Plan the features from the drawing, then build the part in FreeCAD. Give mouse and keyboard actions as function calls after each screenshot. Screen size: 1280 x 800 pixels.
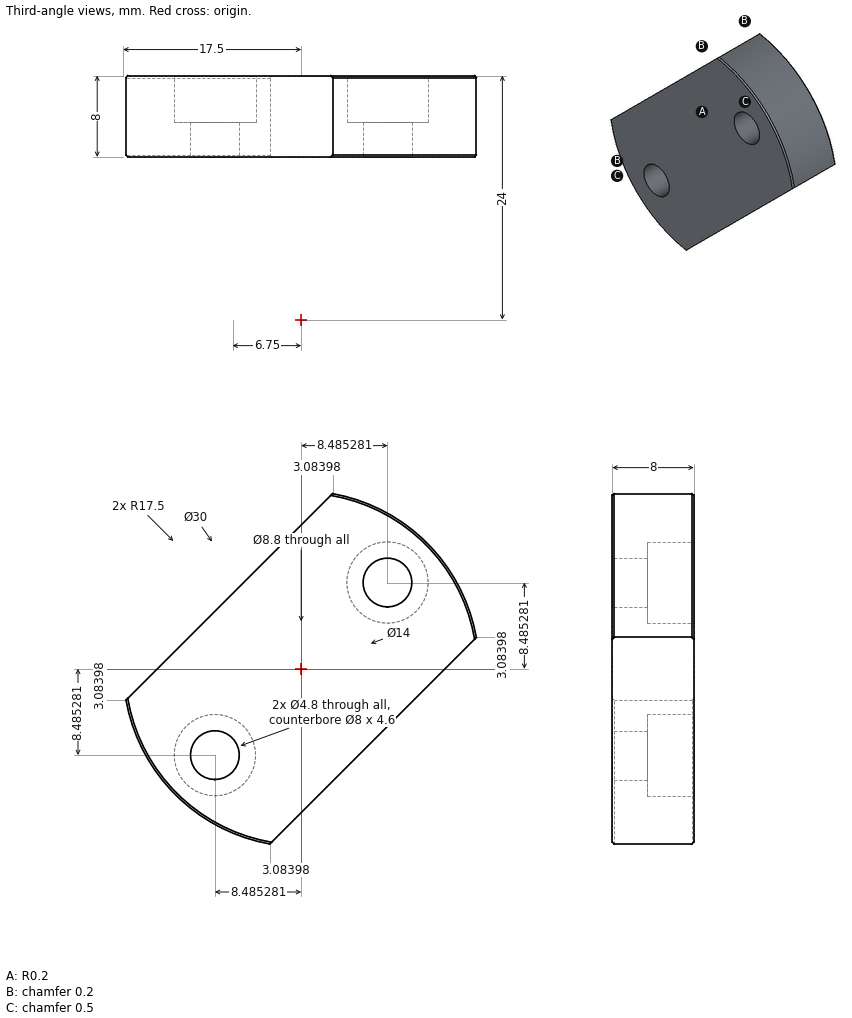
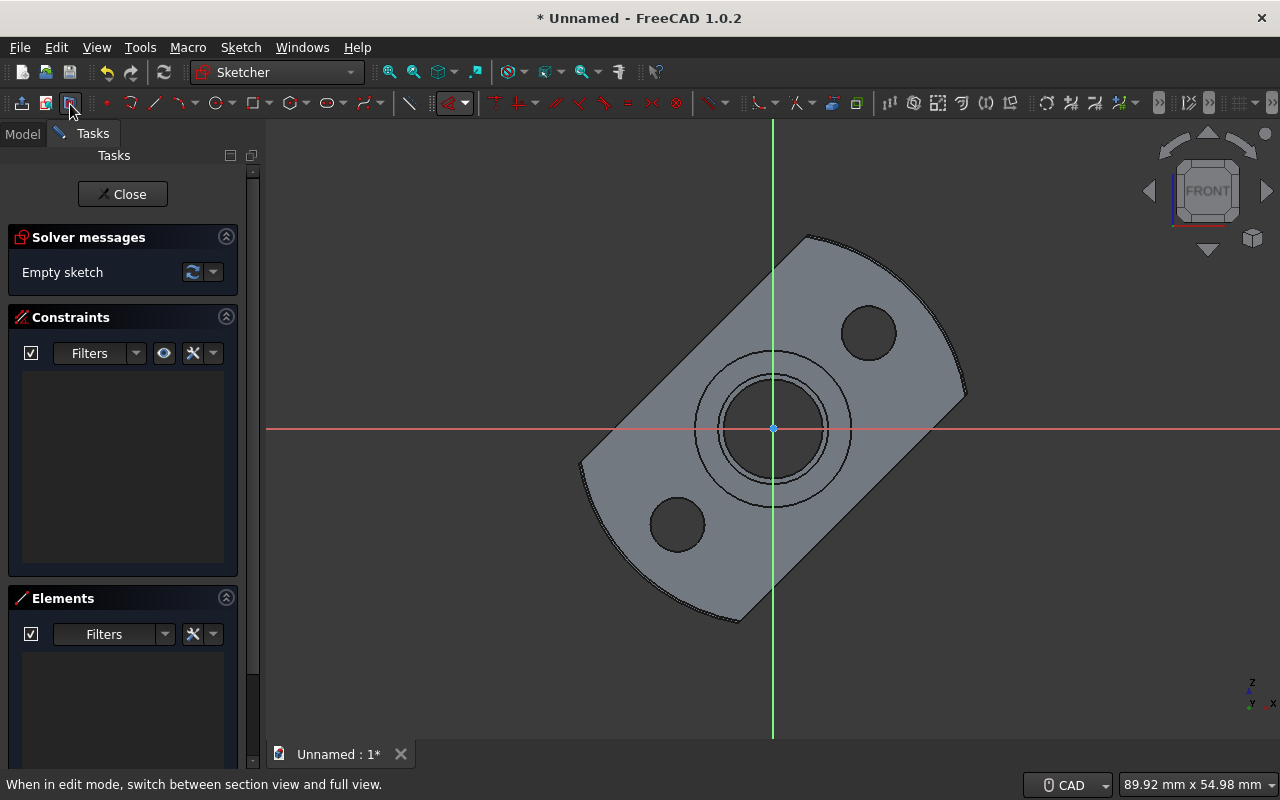
click(216, 104)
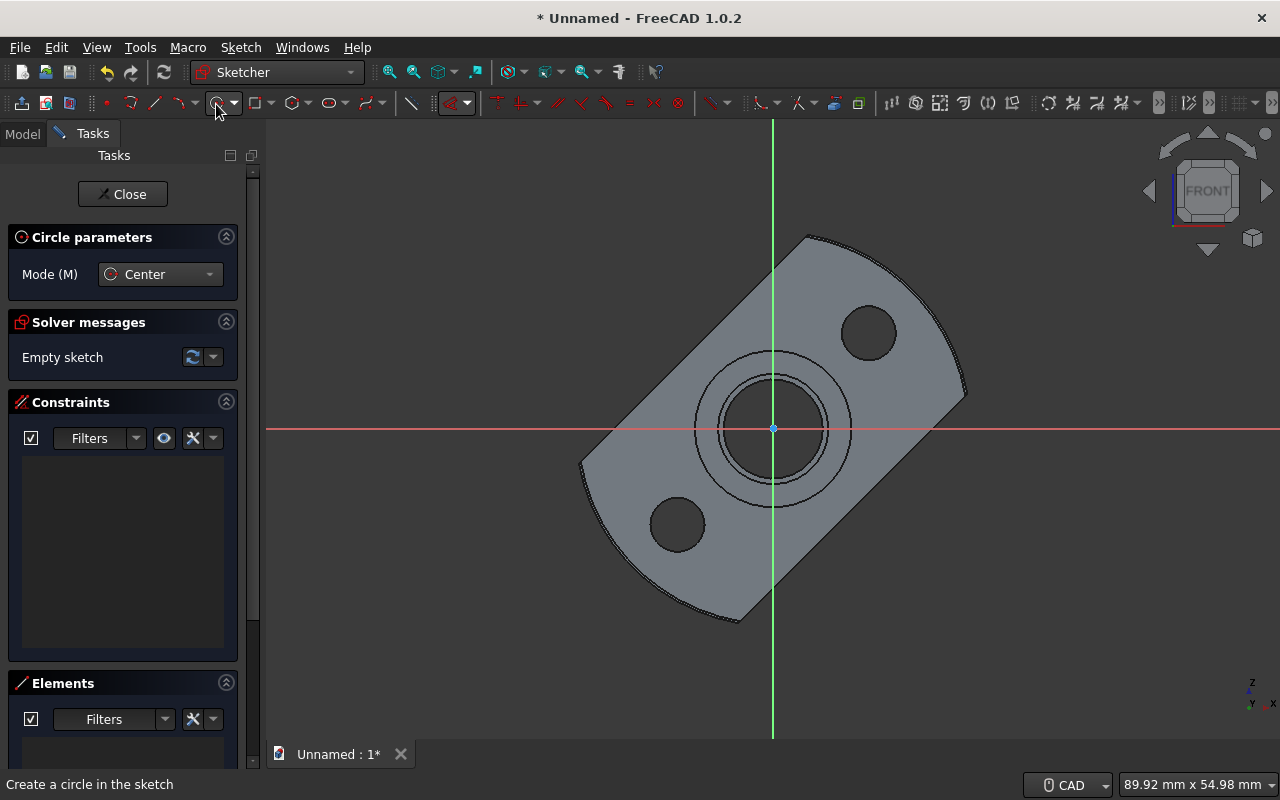
click(773, 429)
move(893, 309)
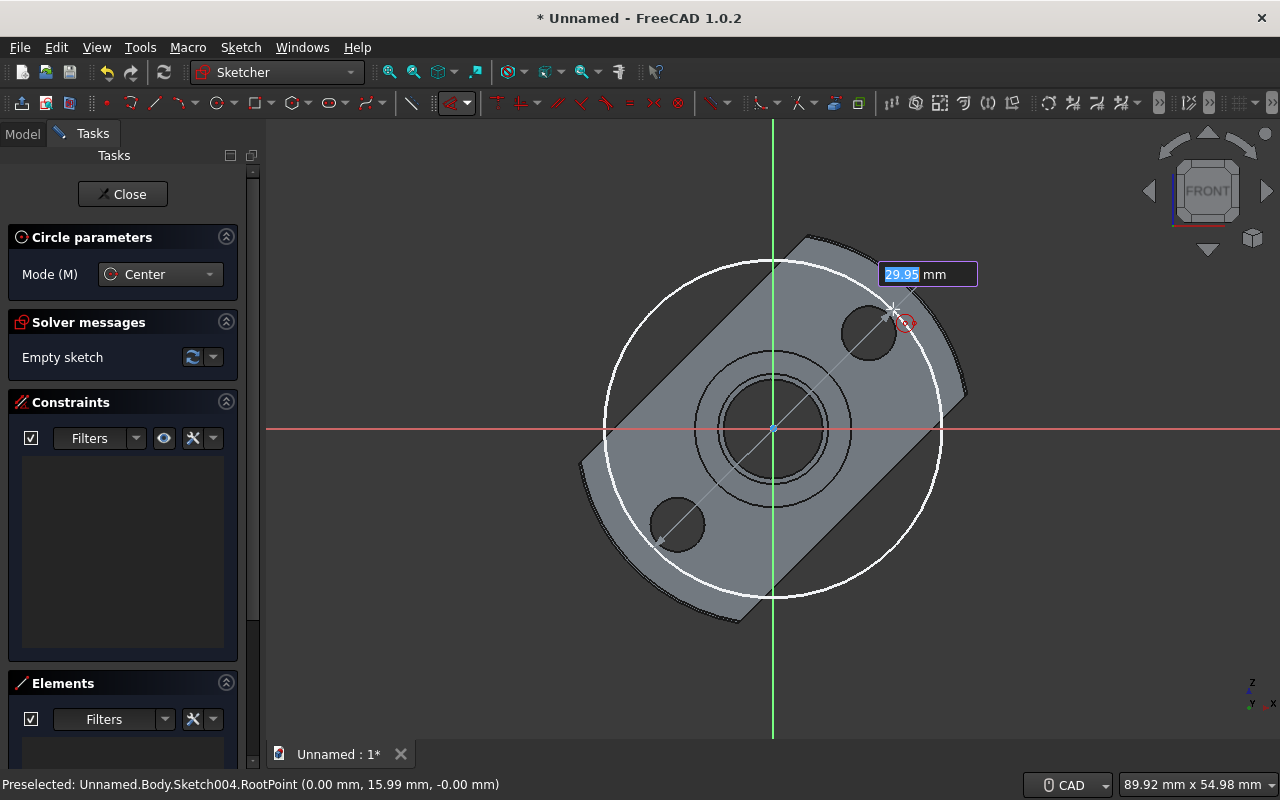
text(30)
key(Return)
key(Escape)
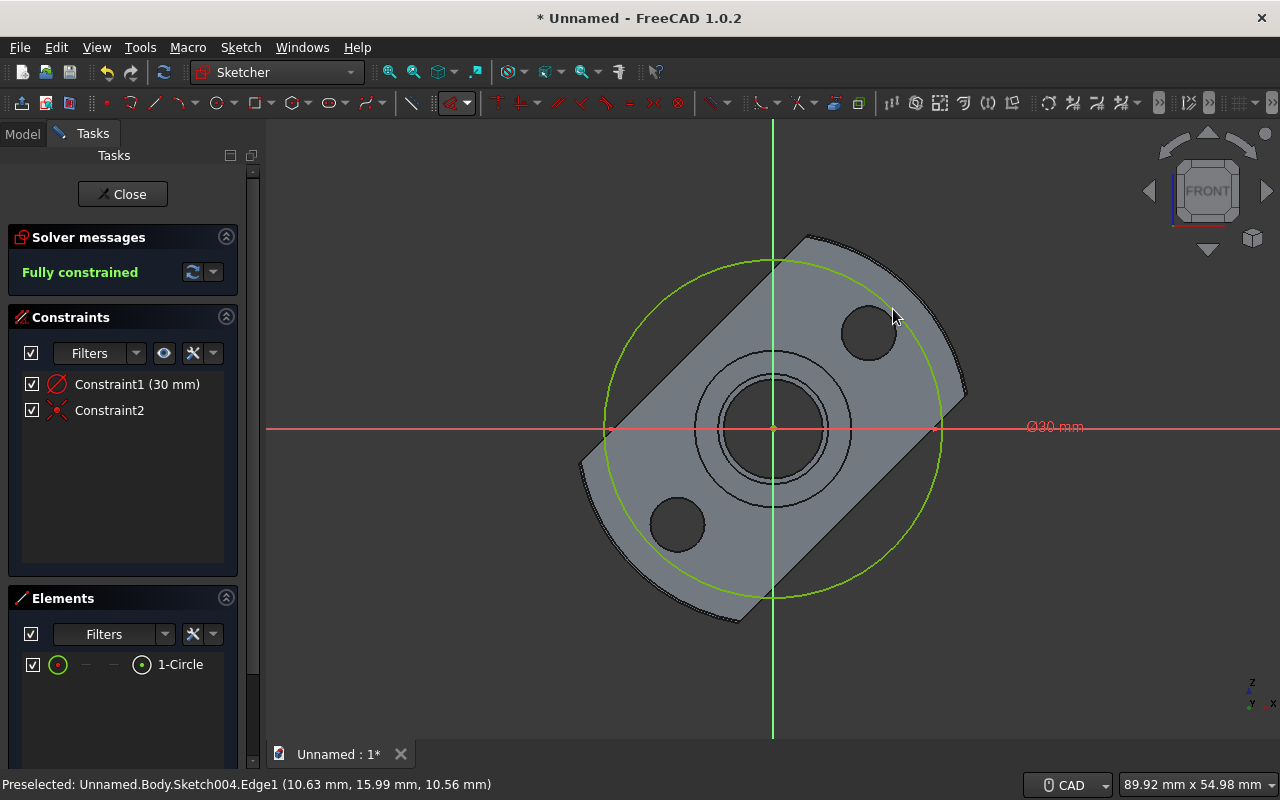
click(123, 194)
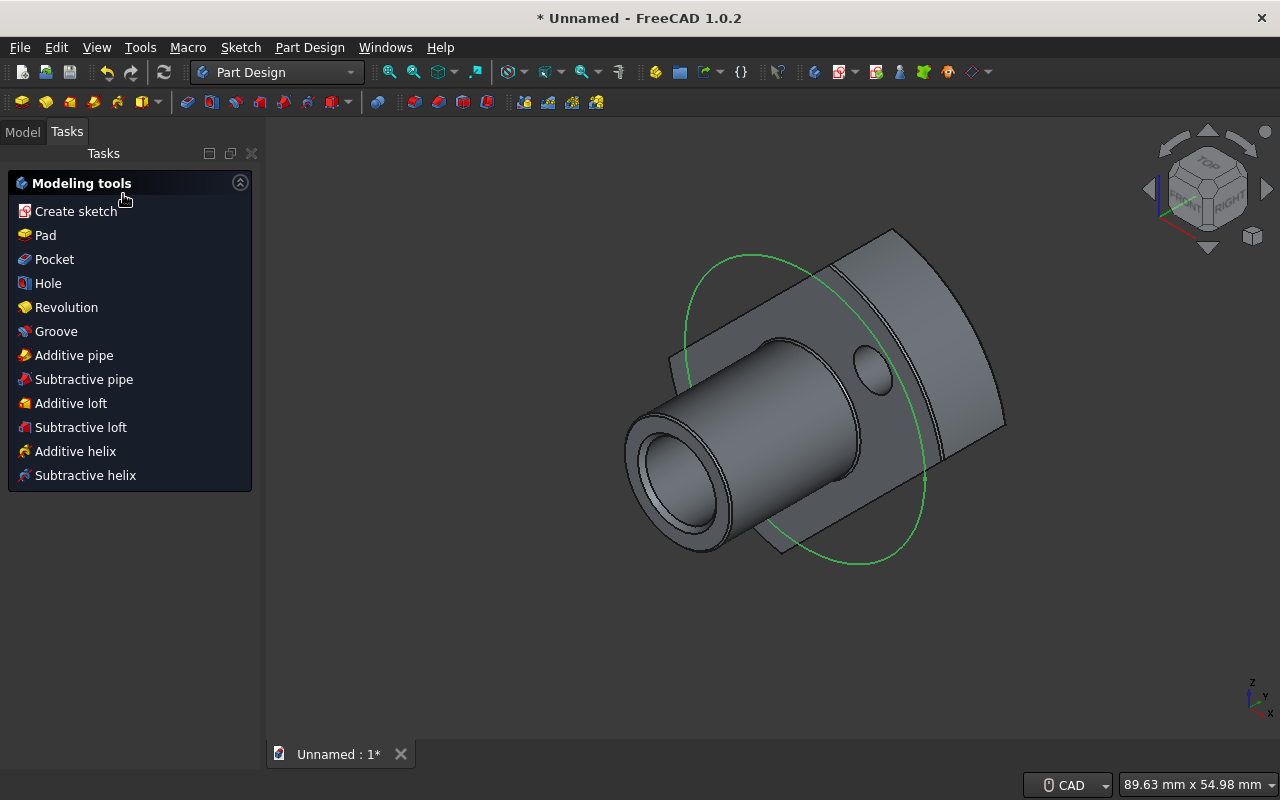
click(188, 102)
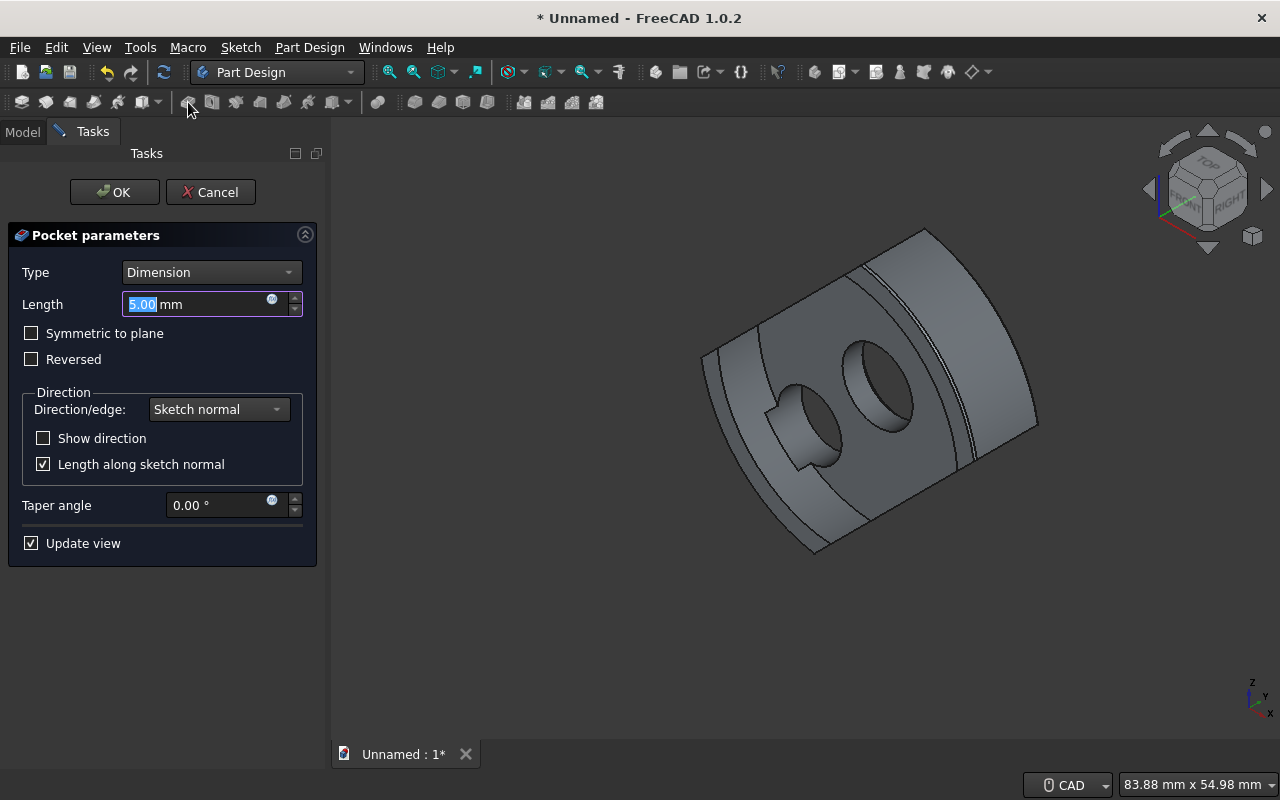
click(212, 272)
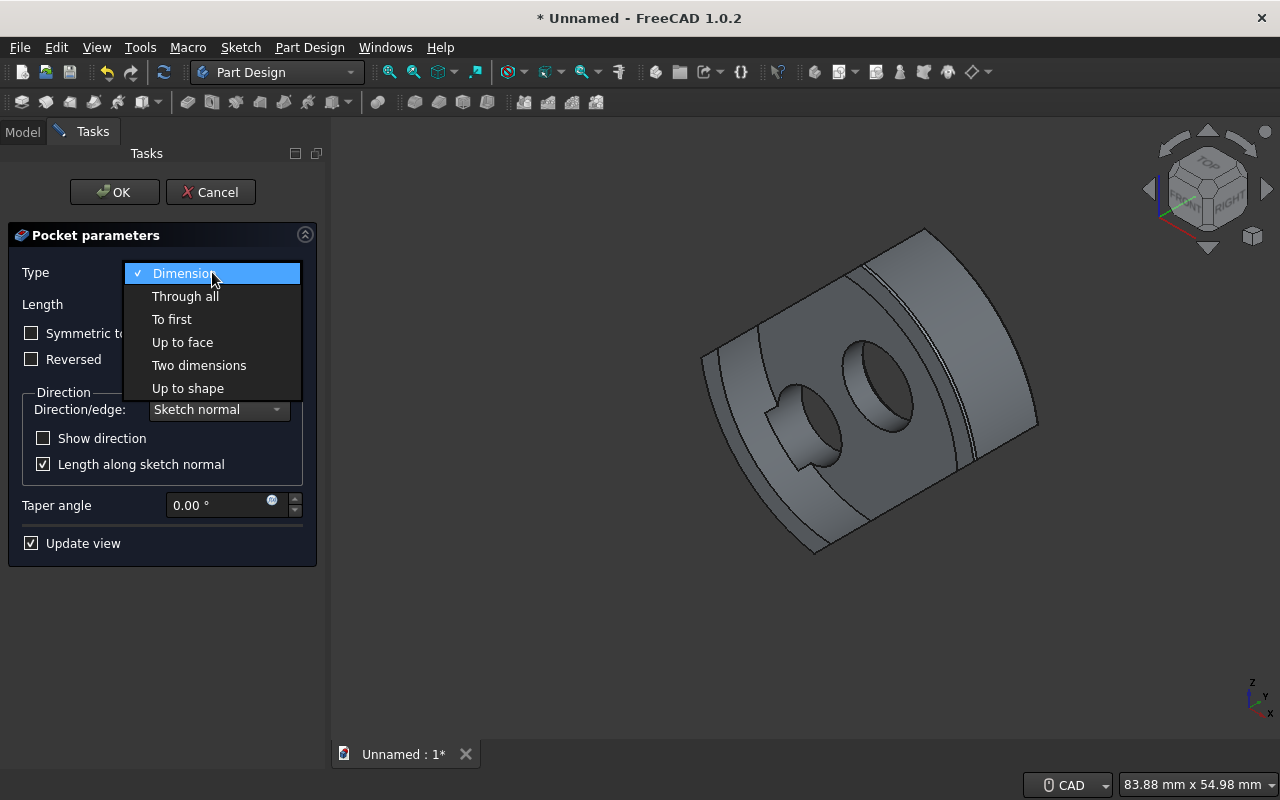
click(212, 296)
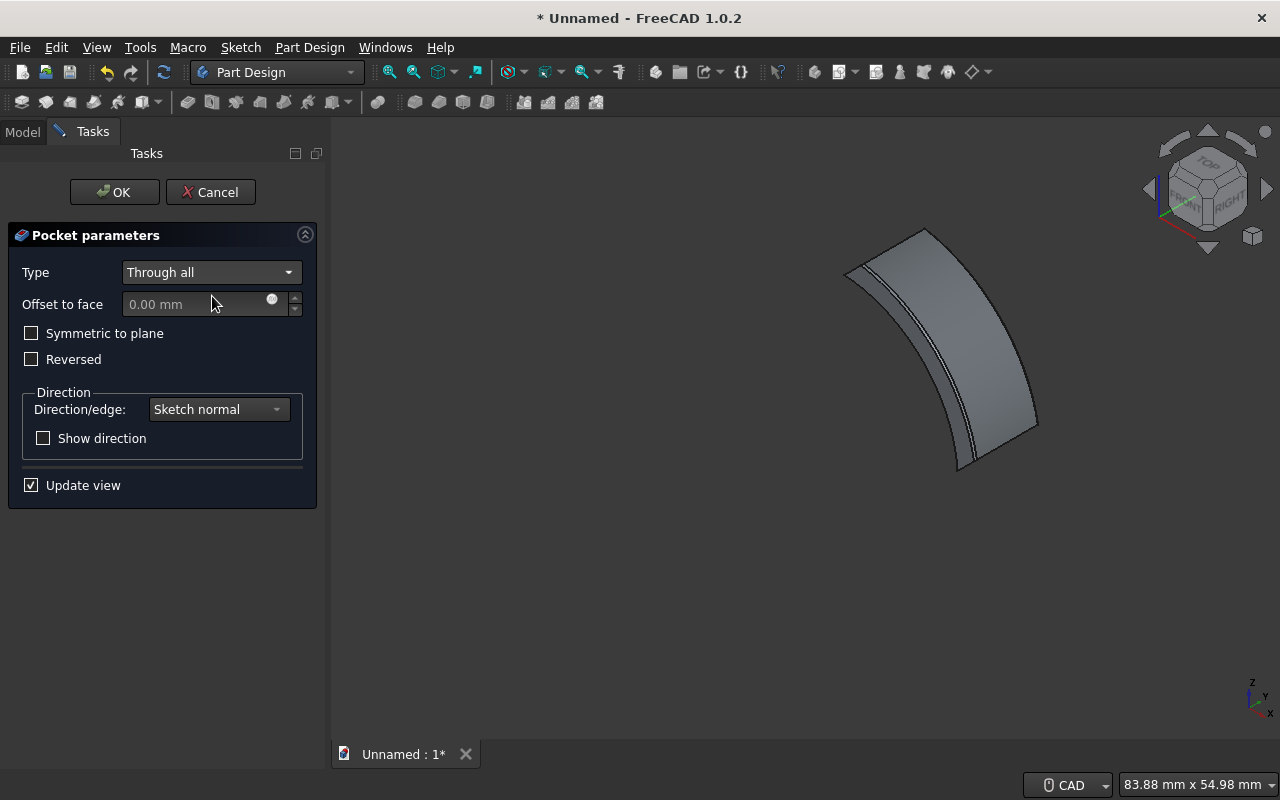
click(30, 359)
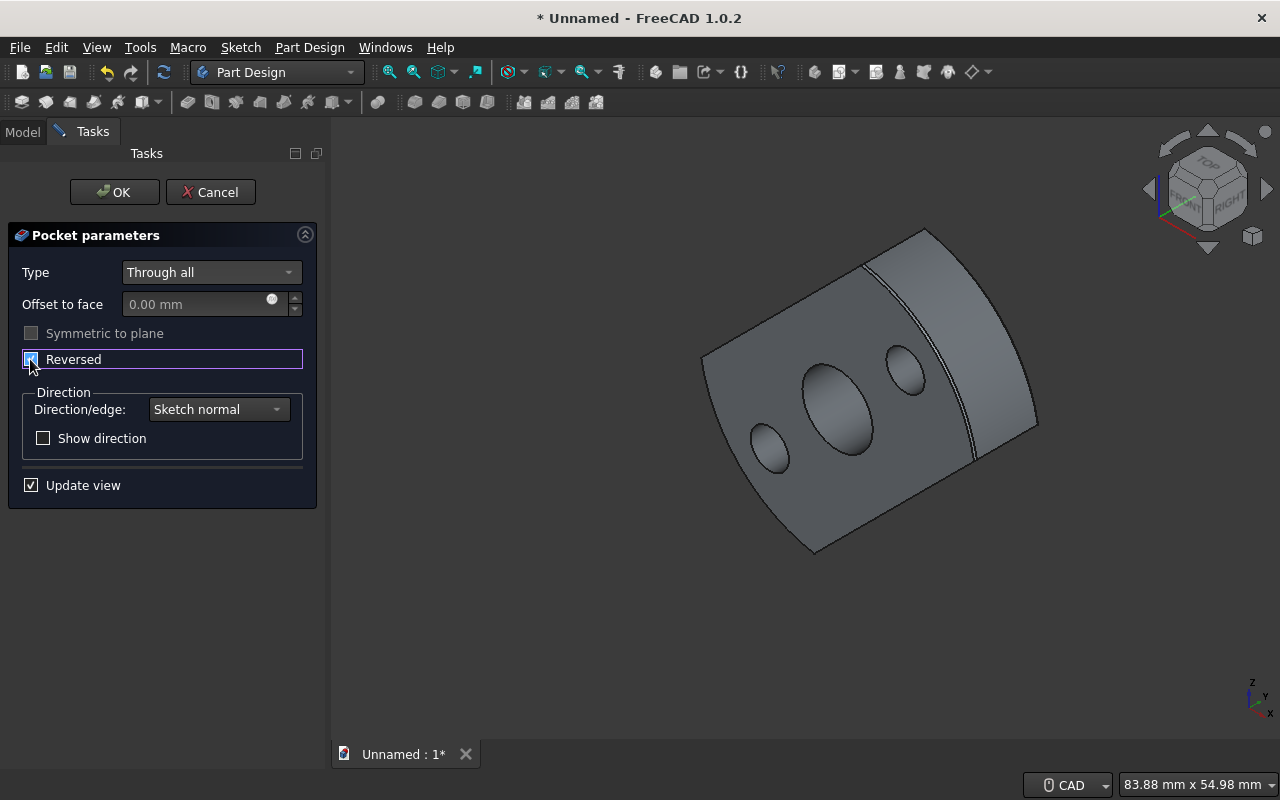
click(115, 192)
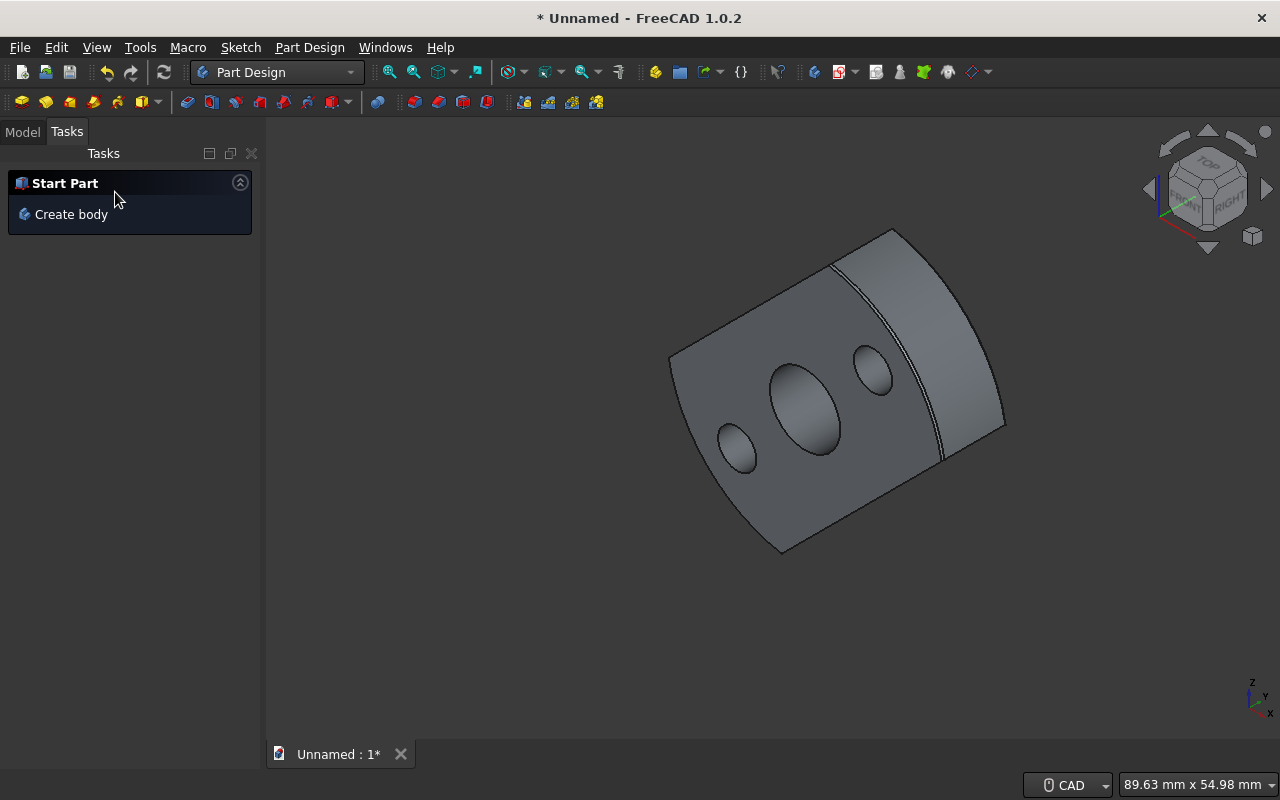
click(883, 454)